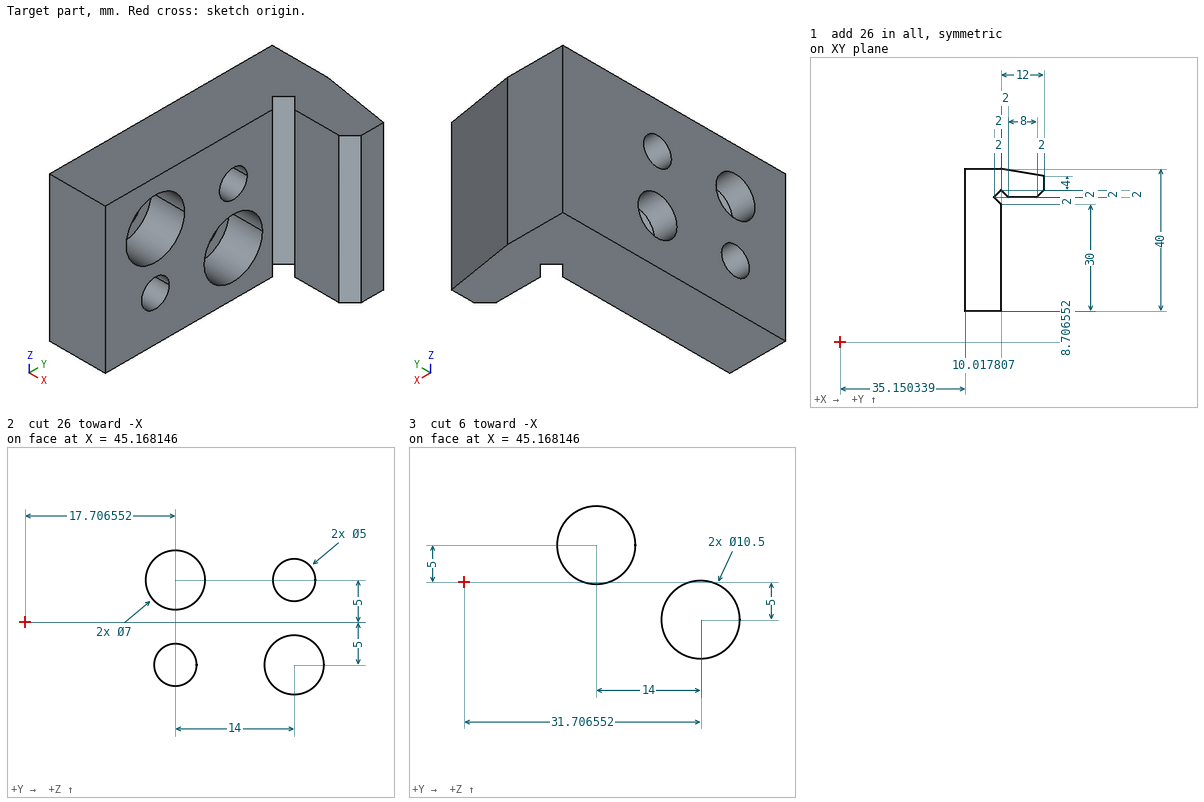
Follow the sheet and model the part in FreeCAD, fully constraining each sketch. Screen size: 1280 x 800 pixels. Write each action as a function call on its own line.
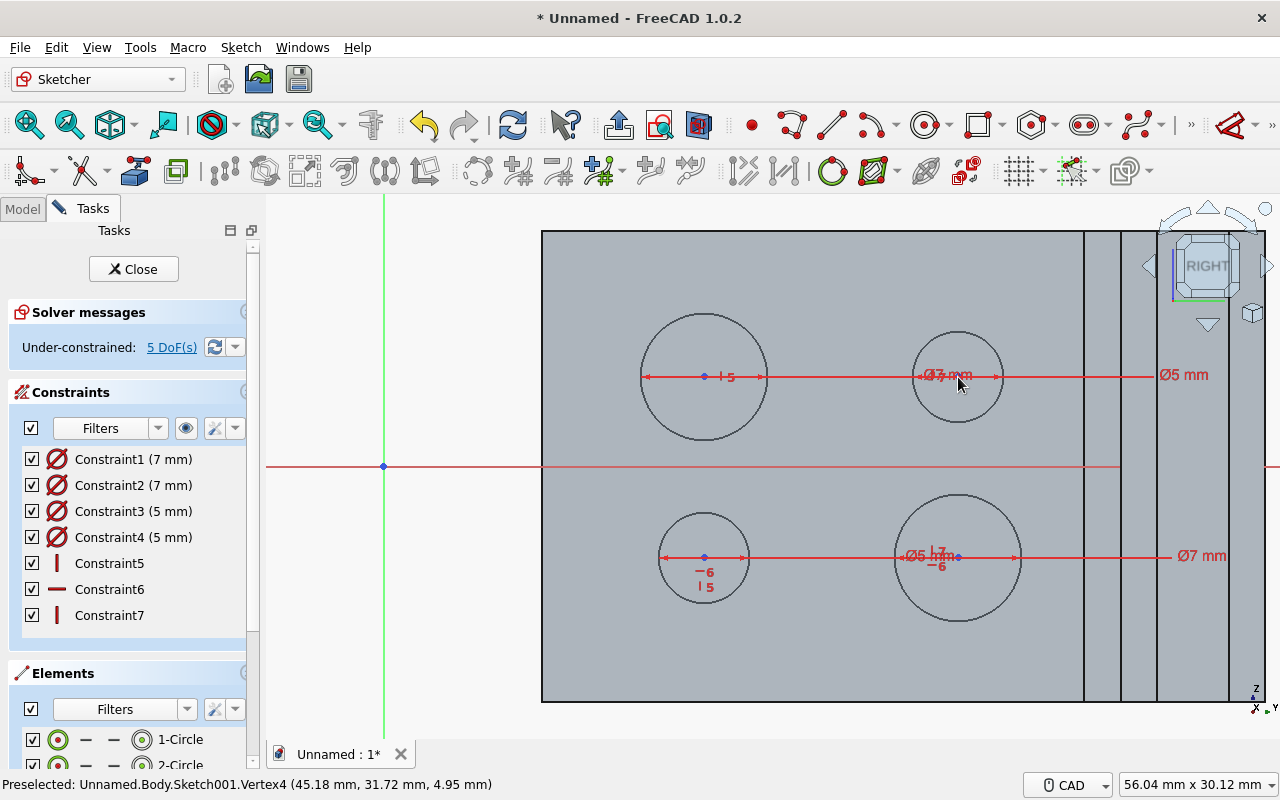
click(704, 377)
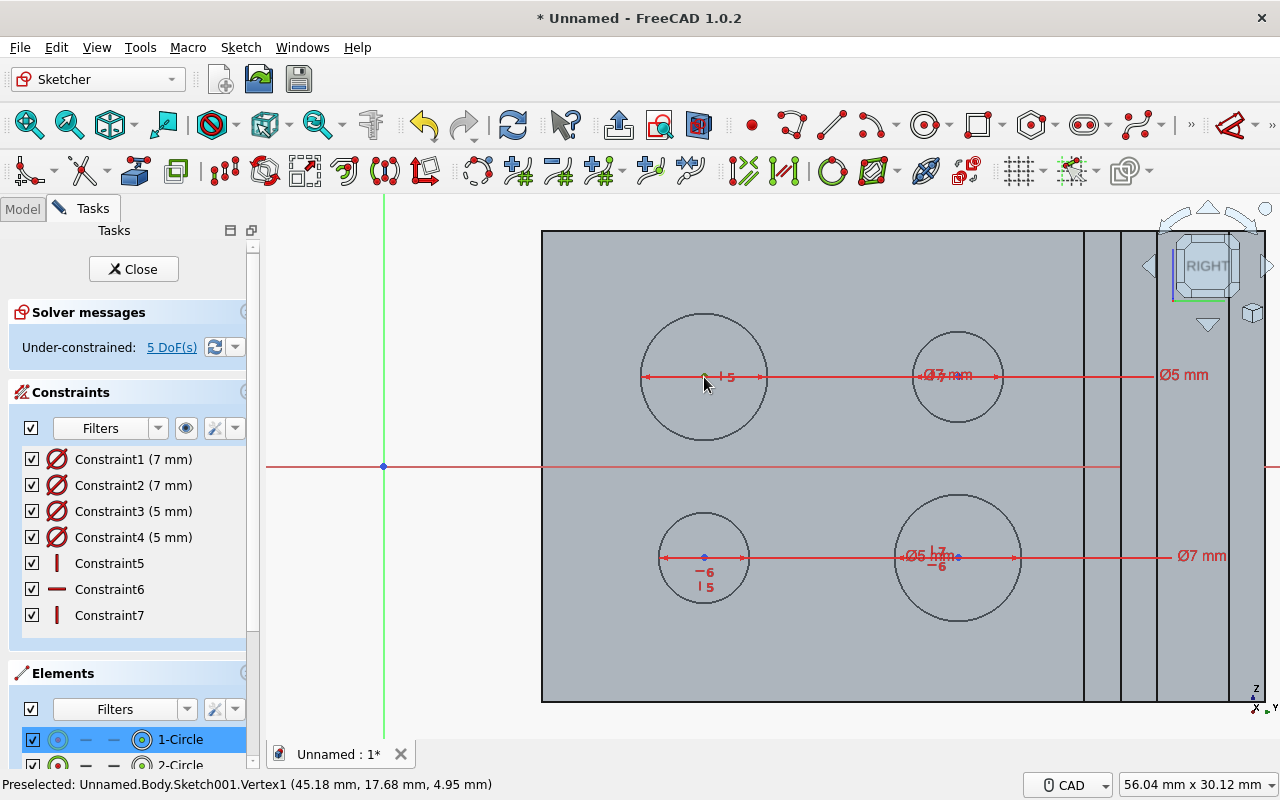
click(958, 377)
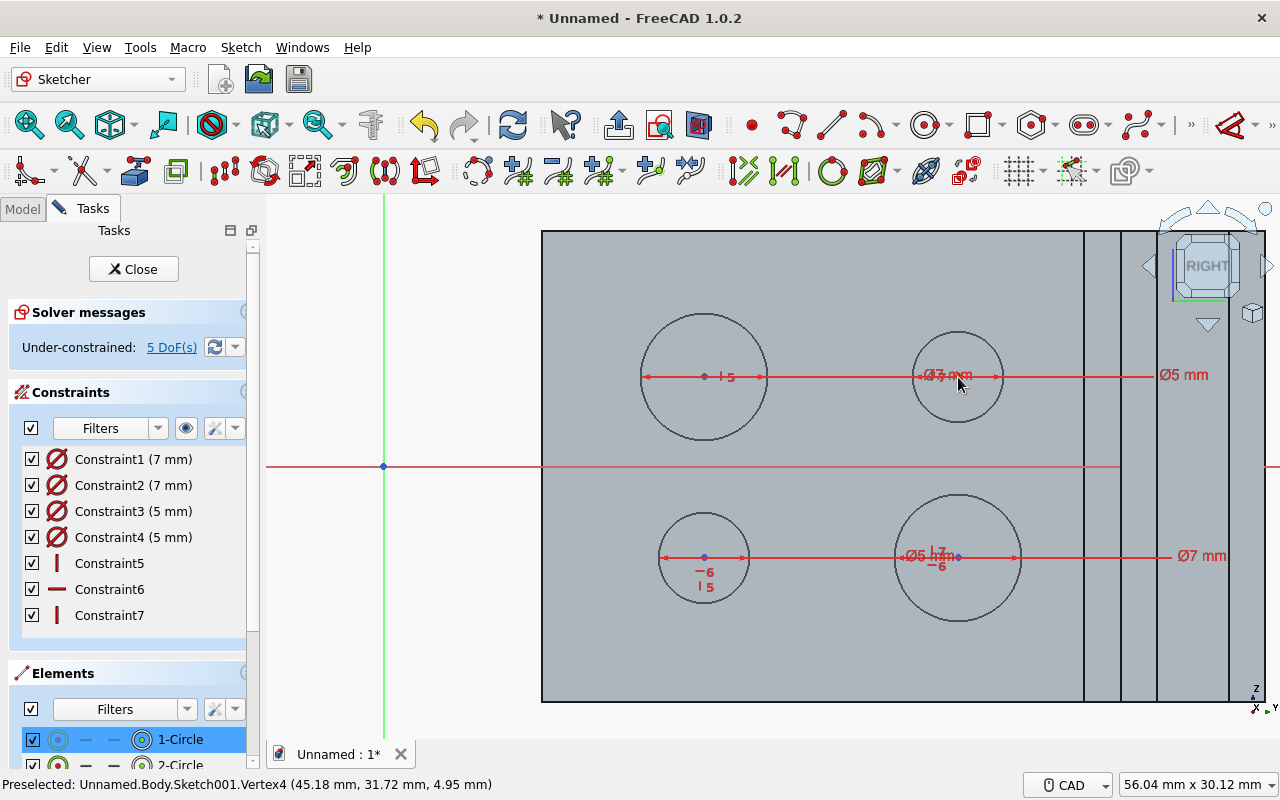
key(h)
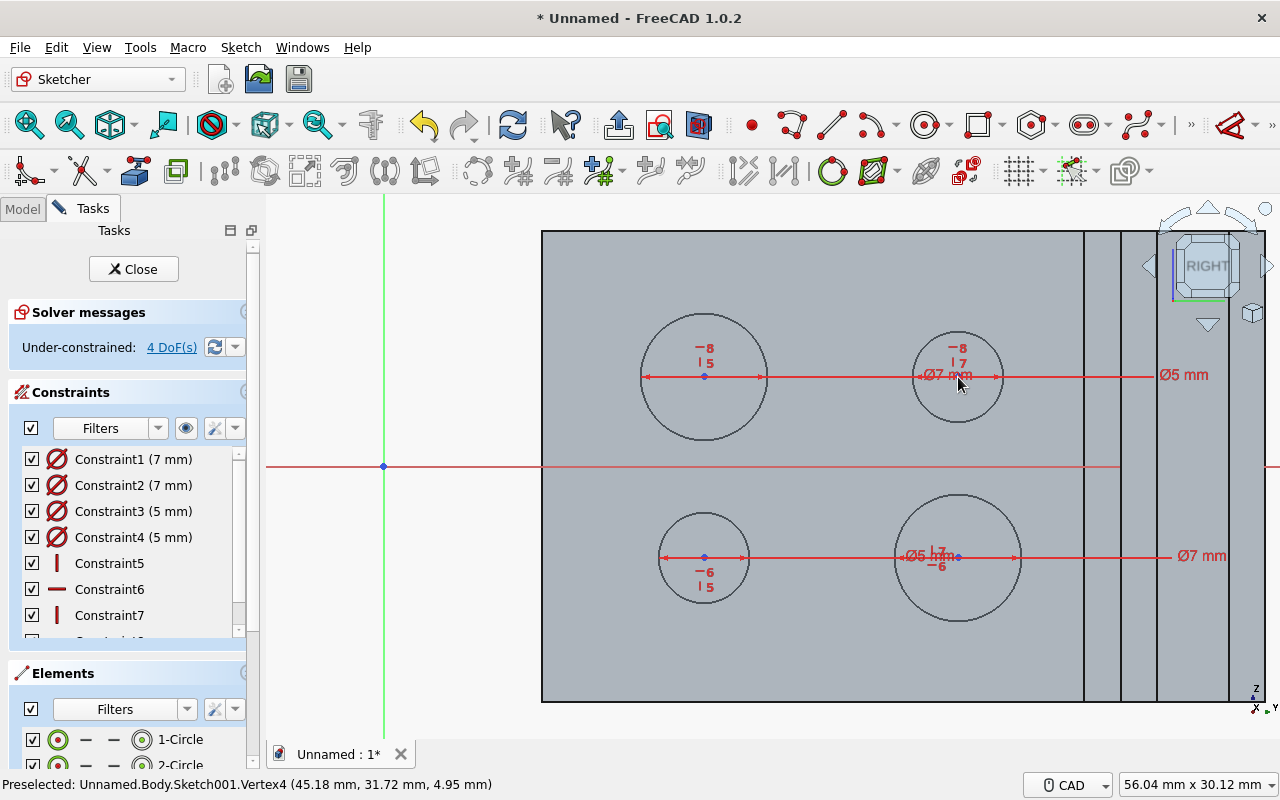
click(1230, 126)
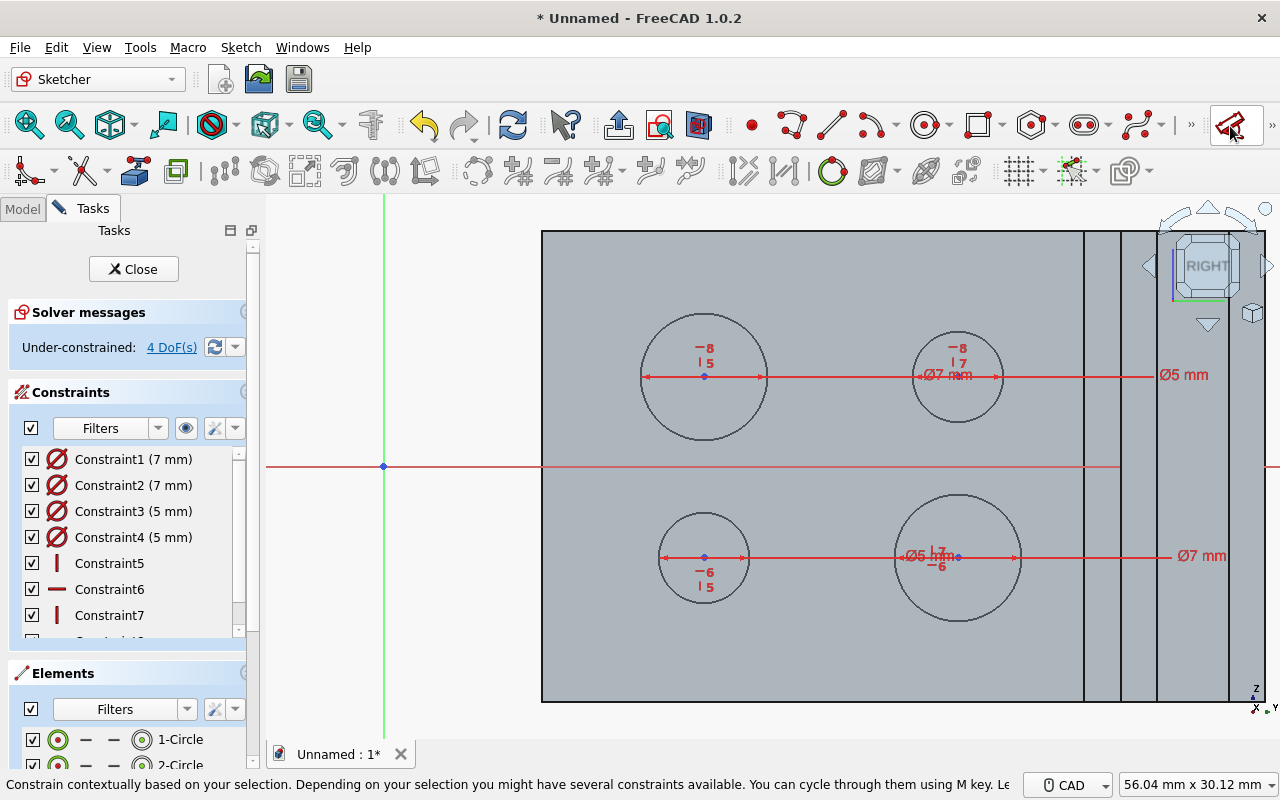
click(704, 377)
click(350, 422)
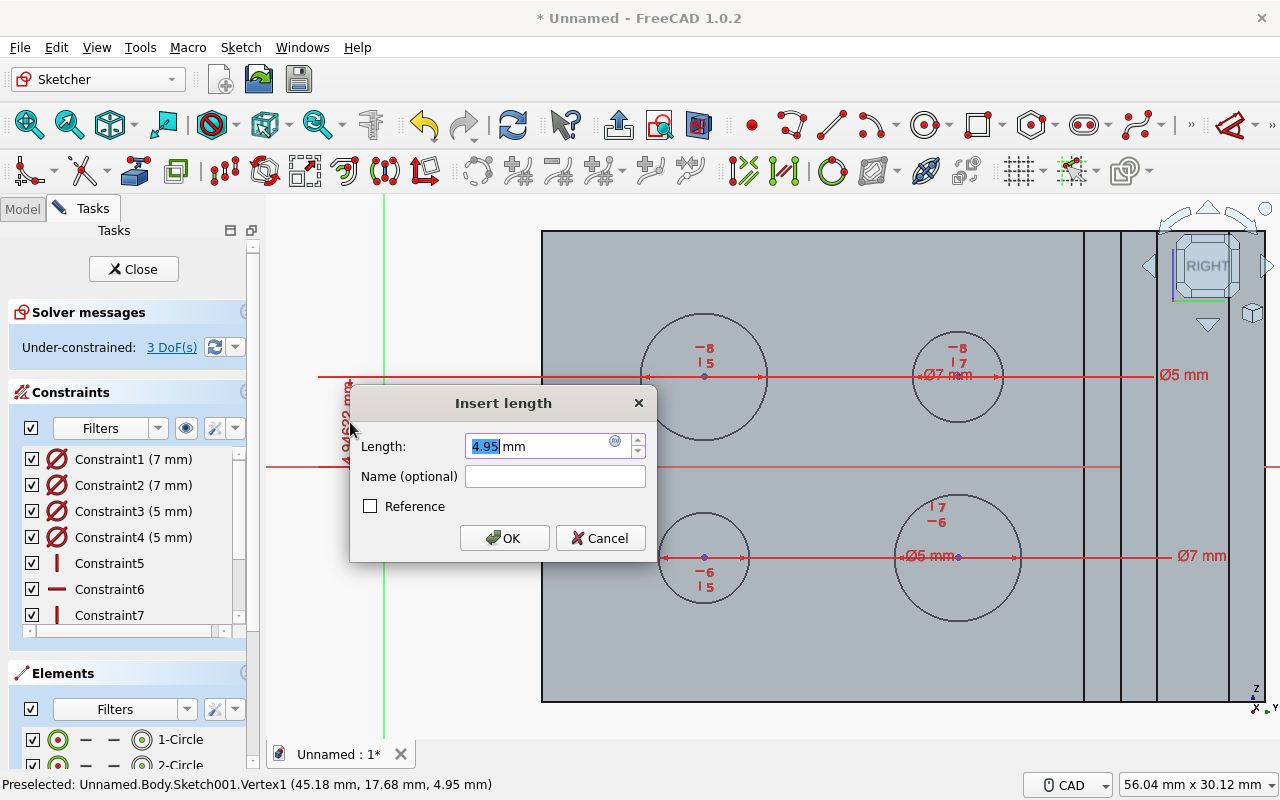
text(5)
key(Return)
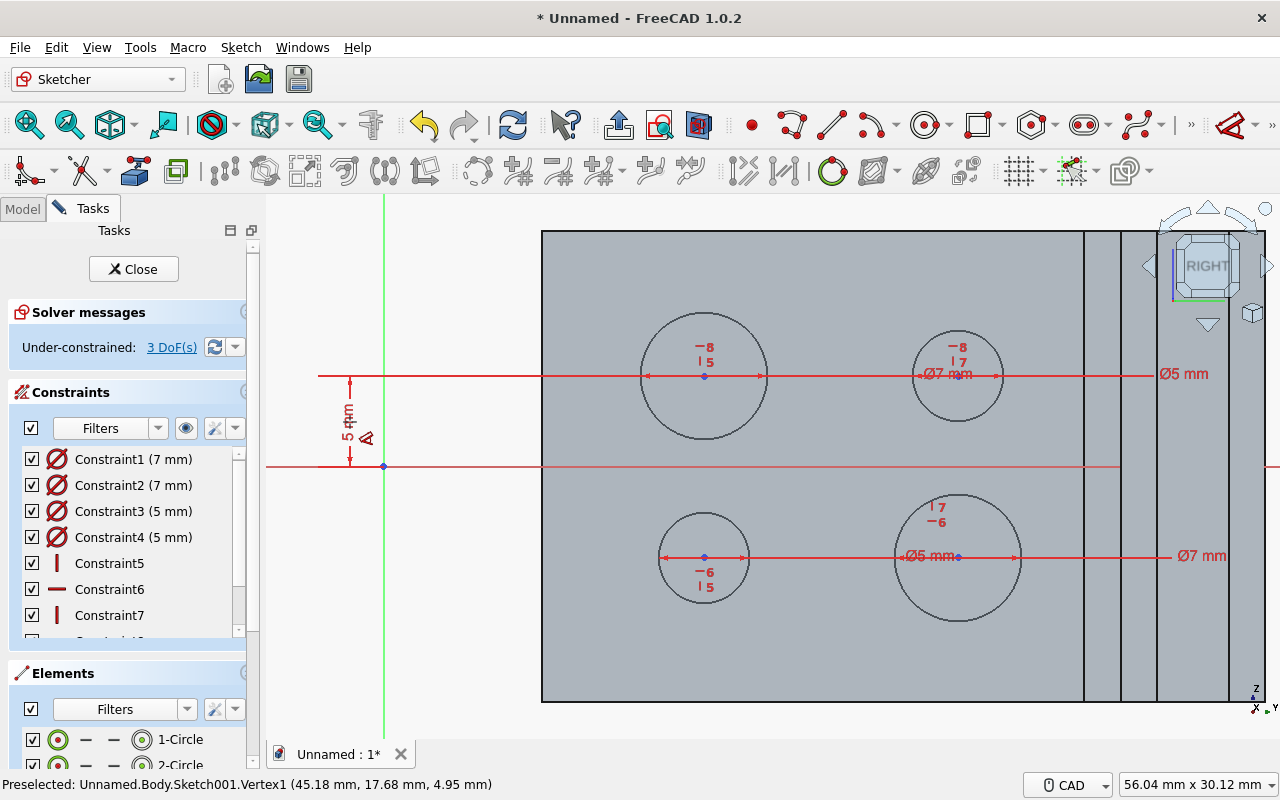
click(958, 558)
click(350, 512)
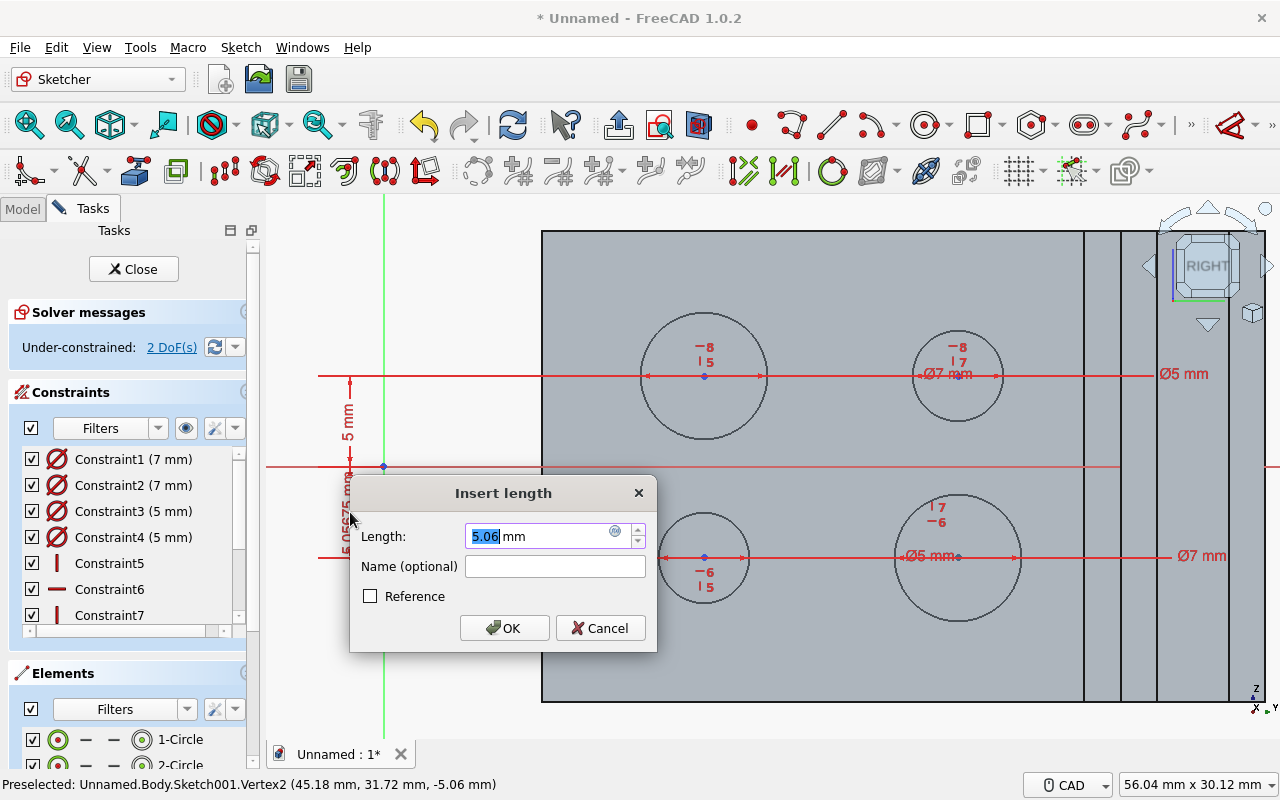
text(5)
key(Return)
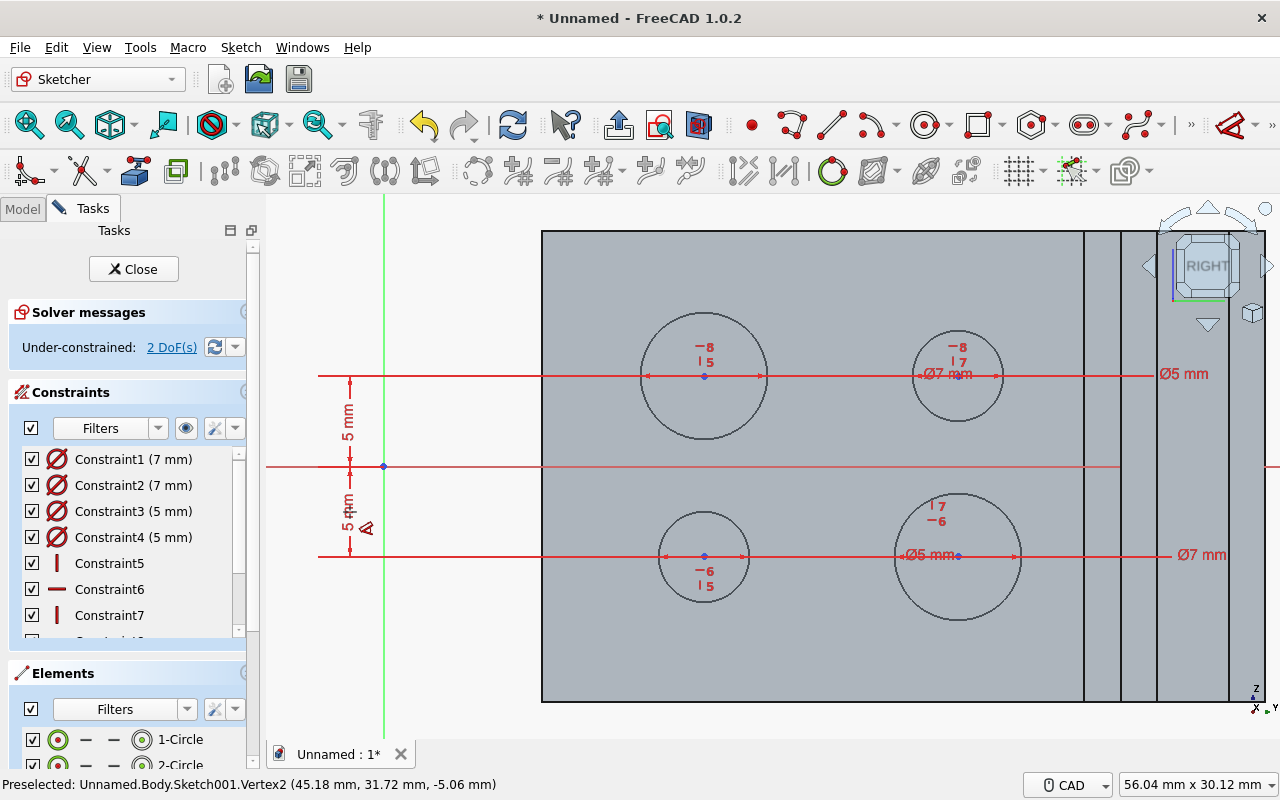
click(704, 376)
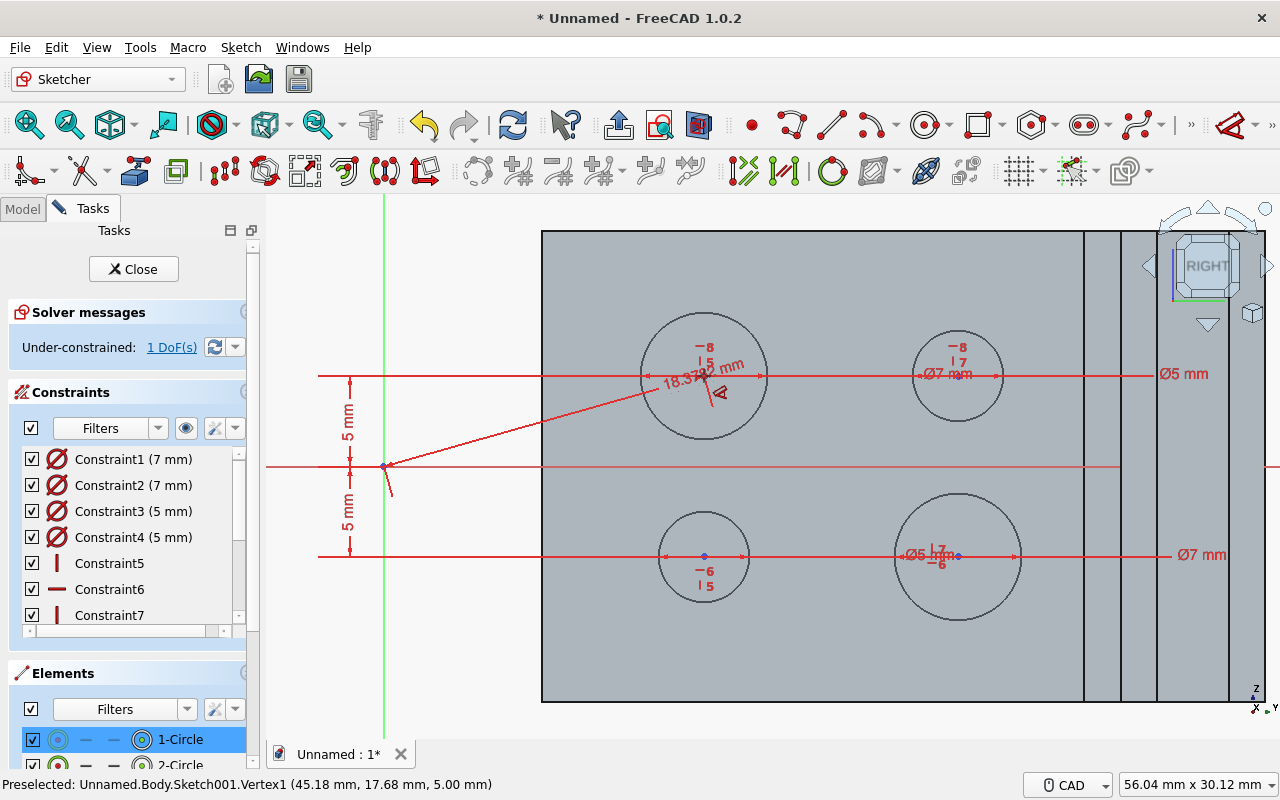
click(958, 557)
click(831, 591)